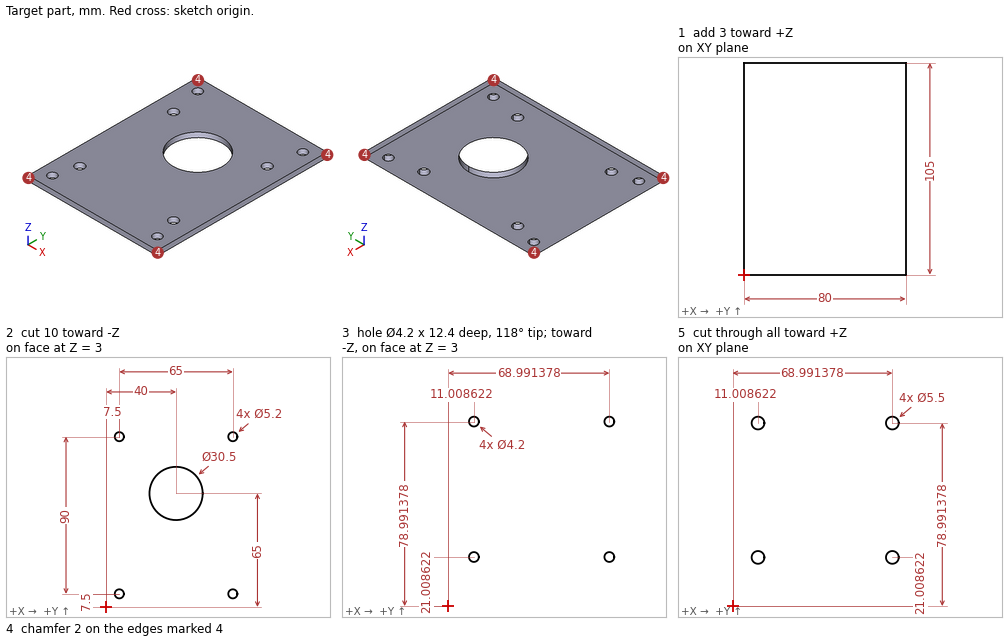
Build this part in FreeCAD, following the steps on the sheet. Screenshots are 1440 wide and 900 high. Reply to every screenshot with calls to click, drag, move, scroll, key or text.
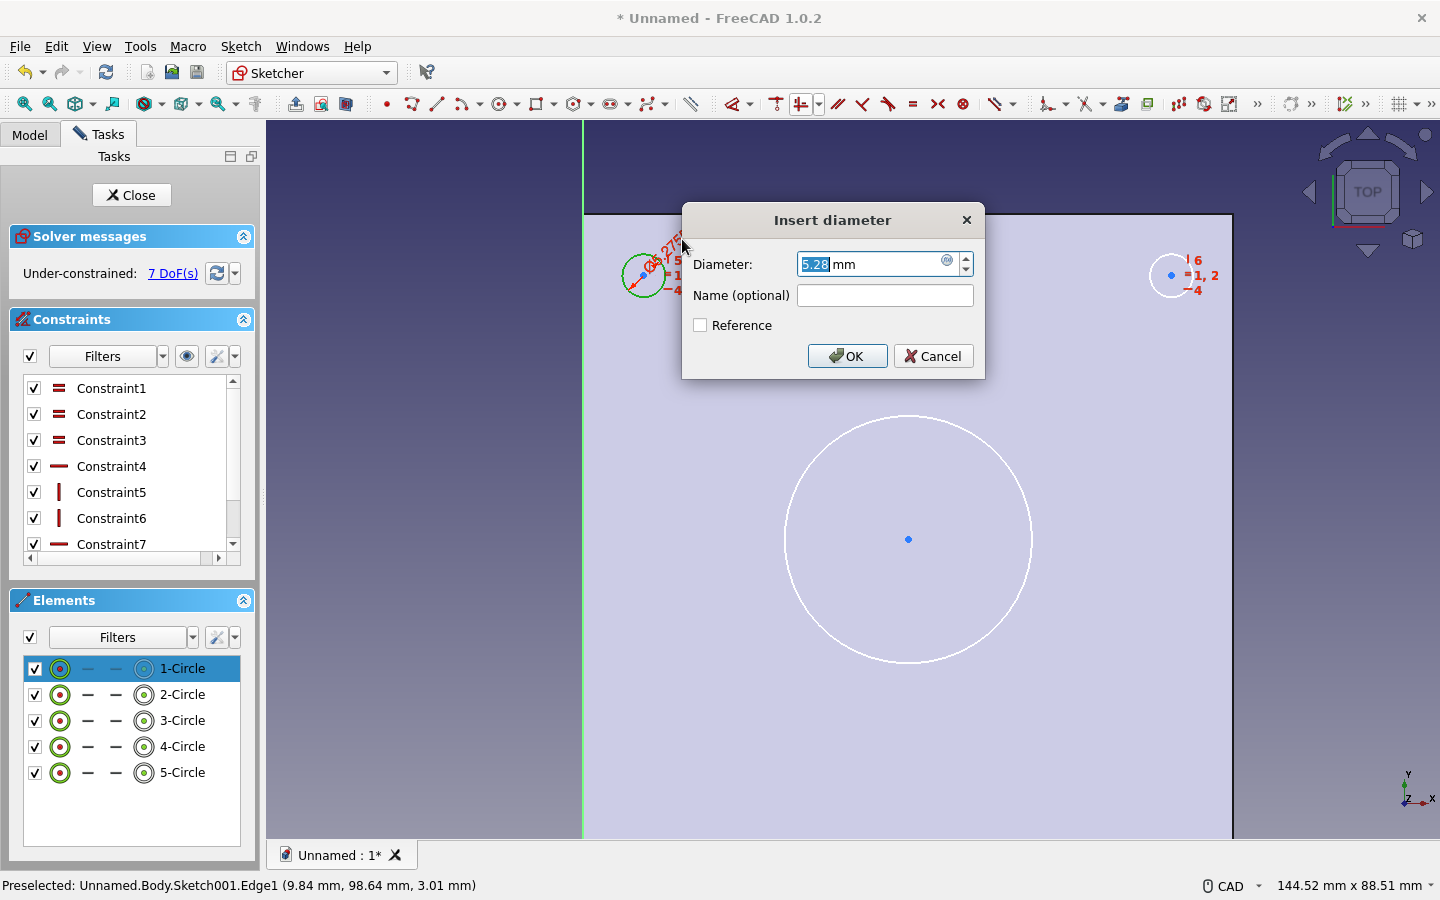
text(5.2)
key(Return)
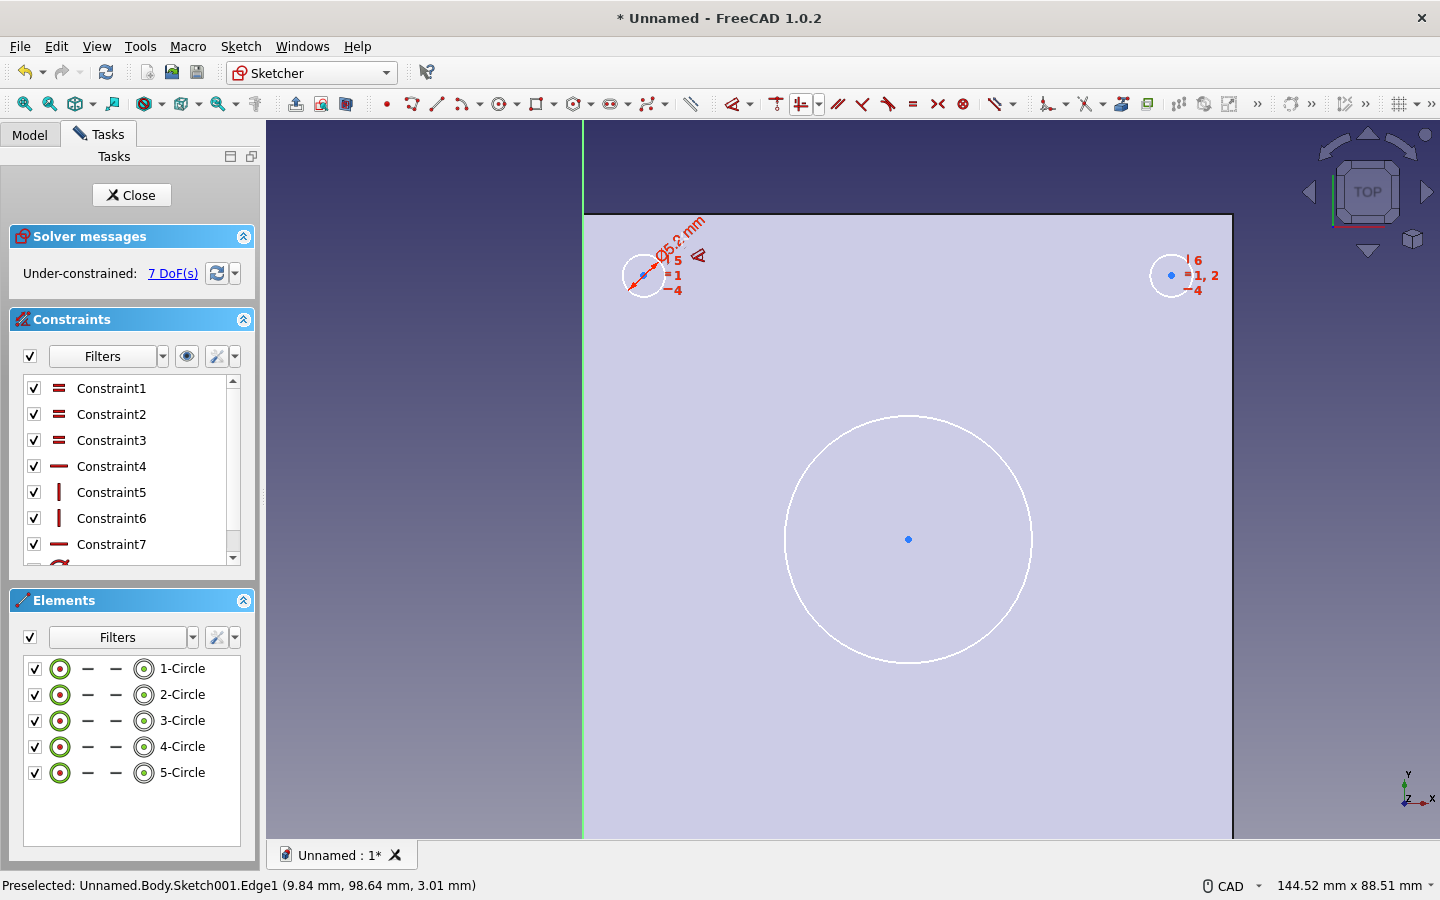
click(996, 452)
click(1019, 429)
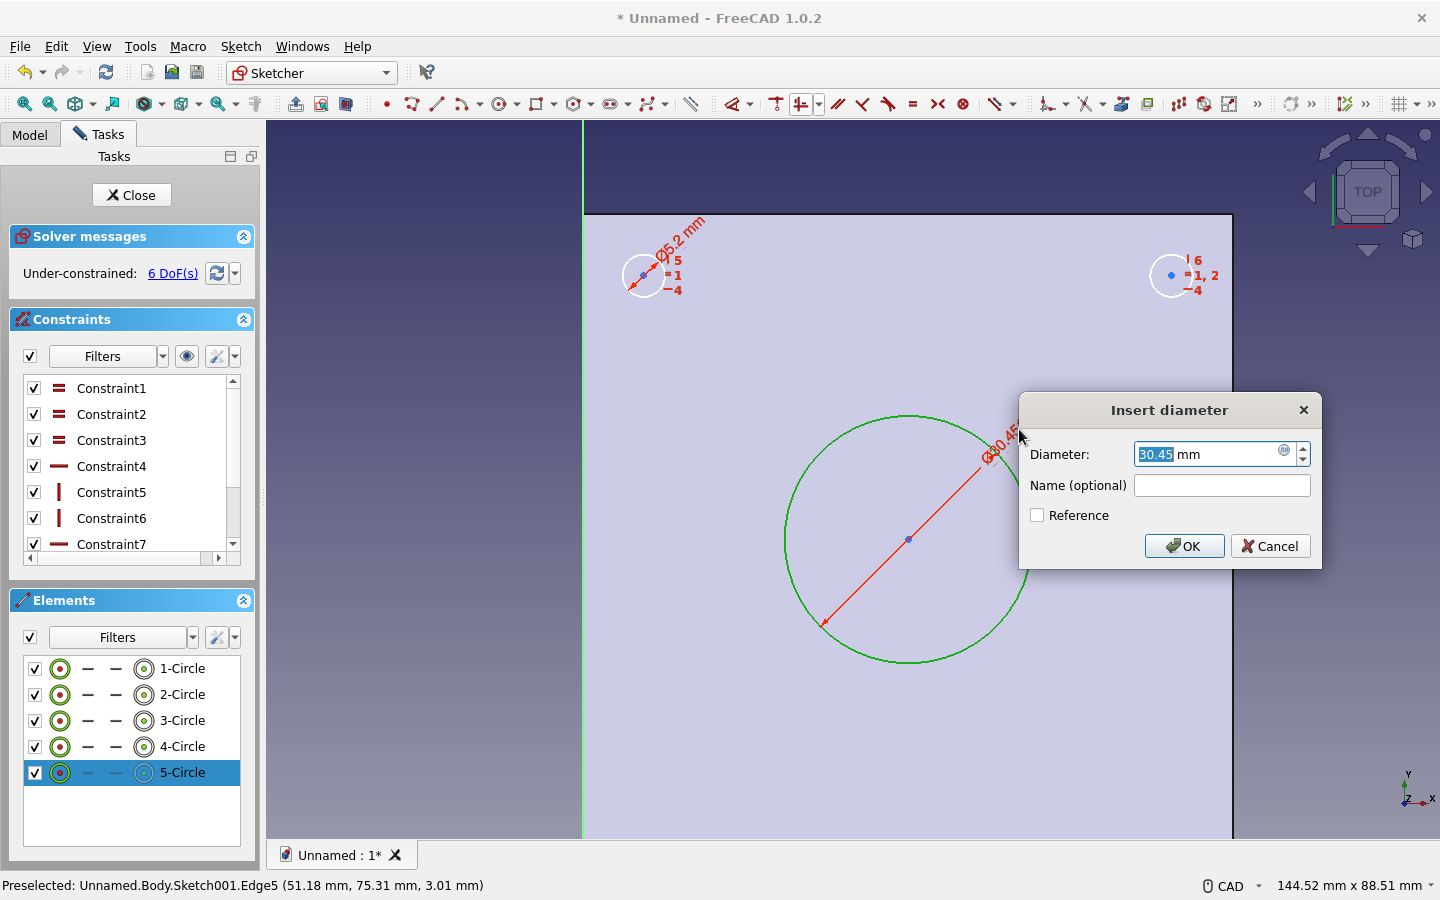
text(30.5)
key(Return)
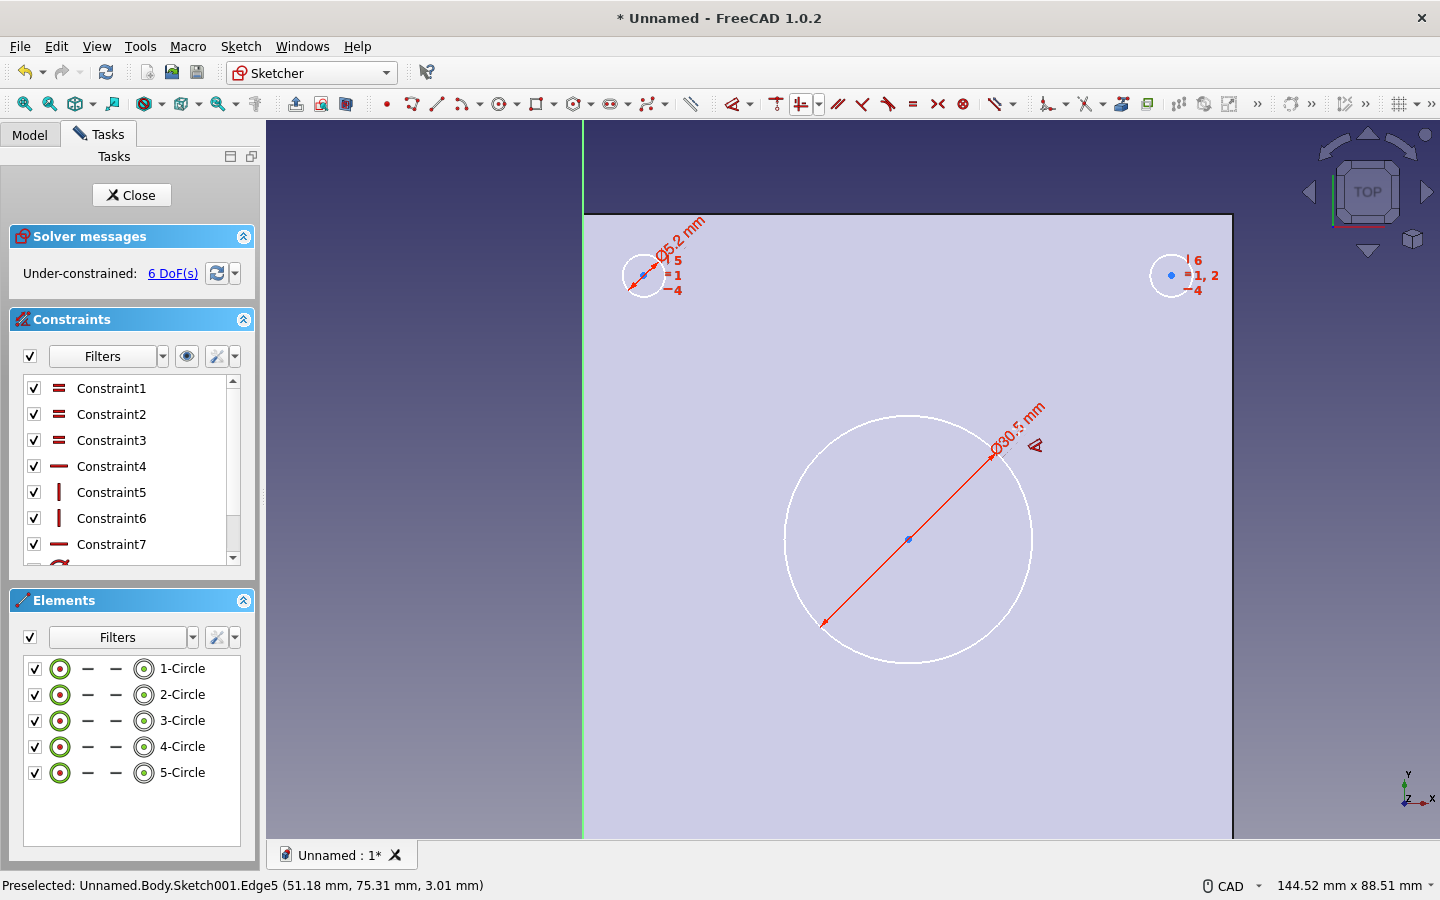
click(908, 540)
click(746, 506)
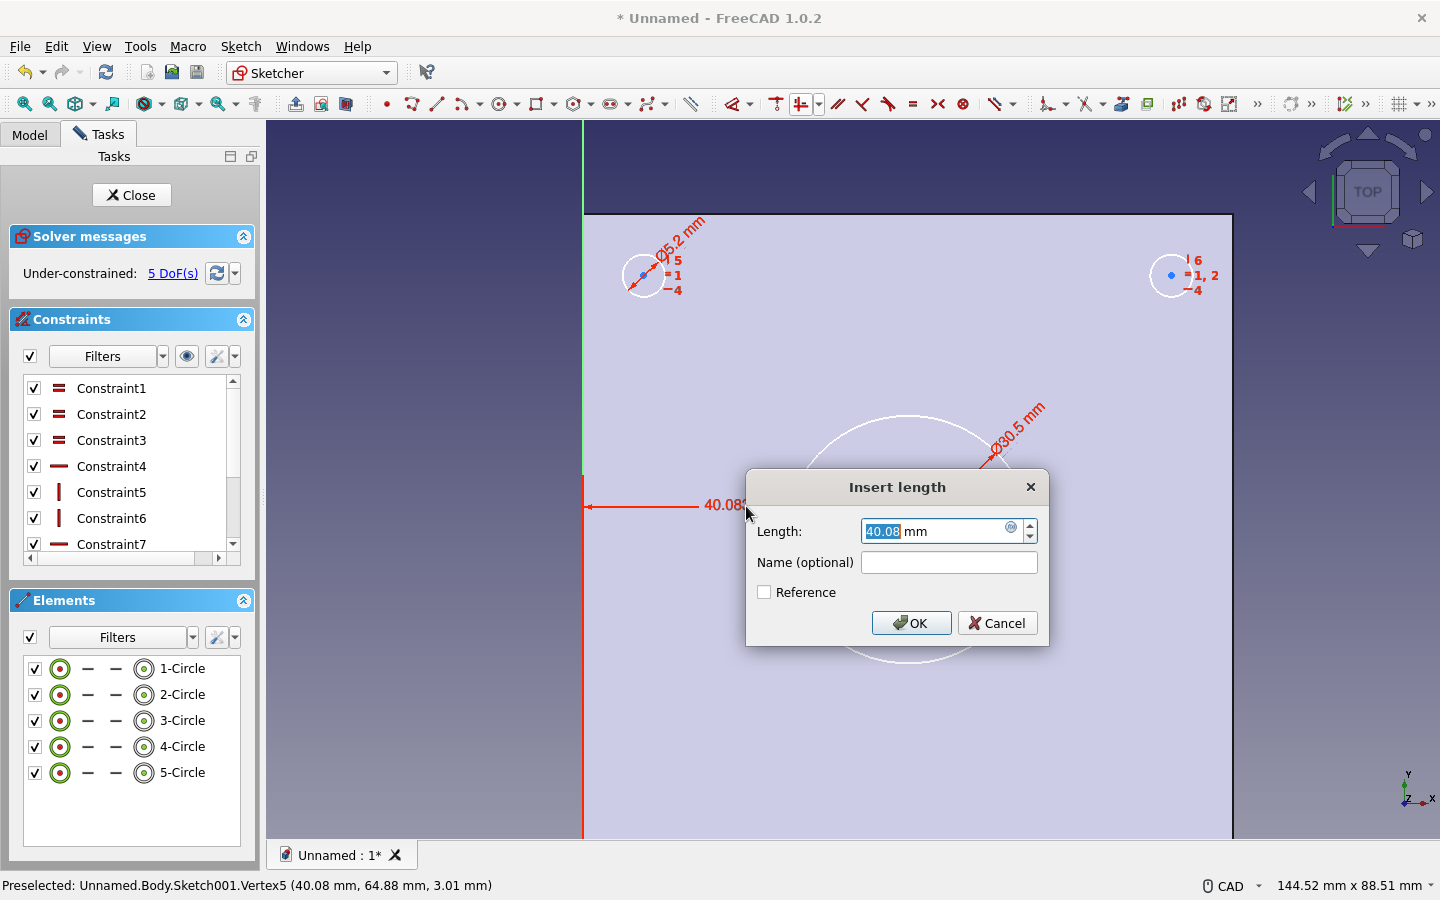
text(40)
key(Return)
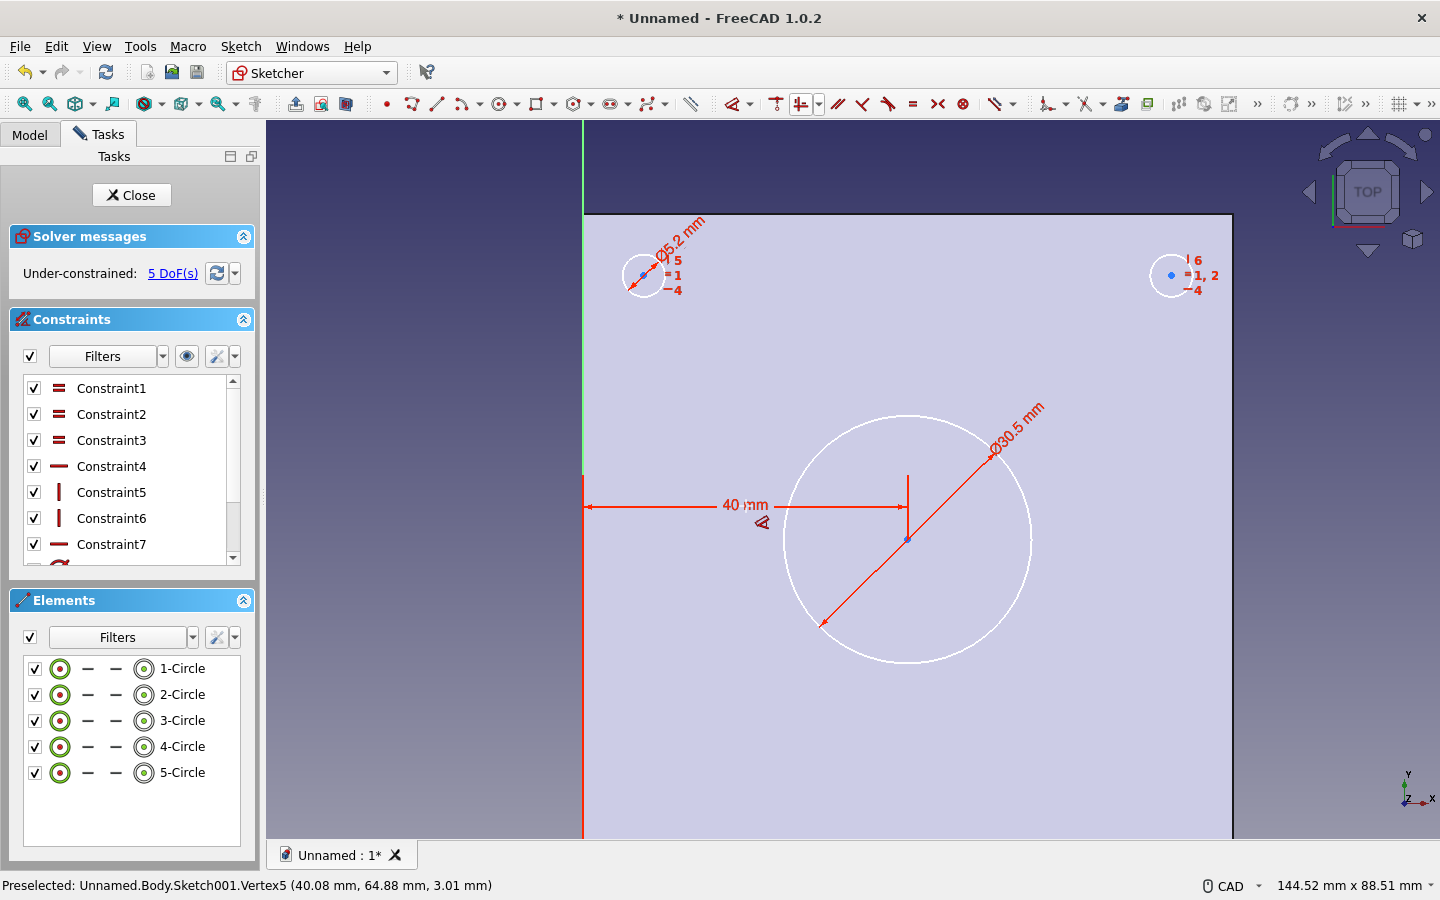
click(908, 540)
click(549, 675)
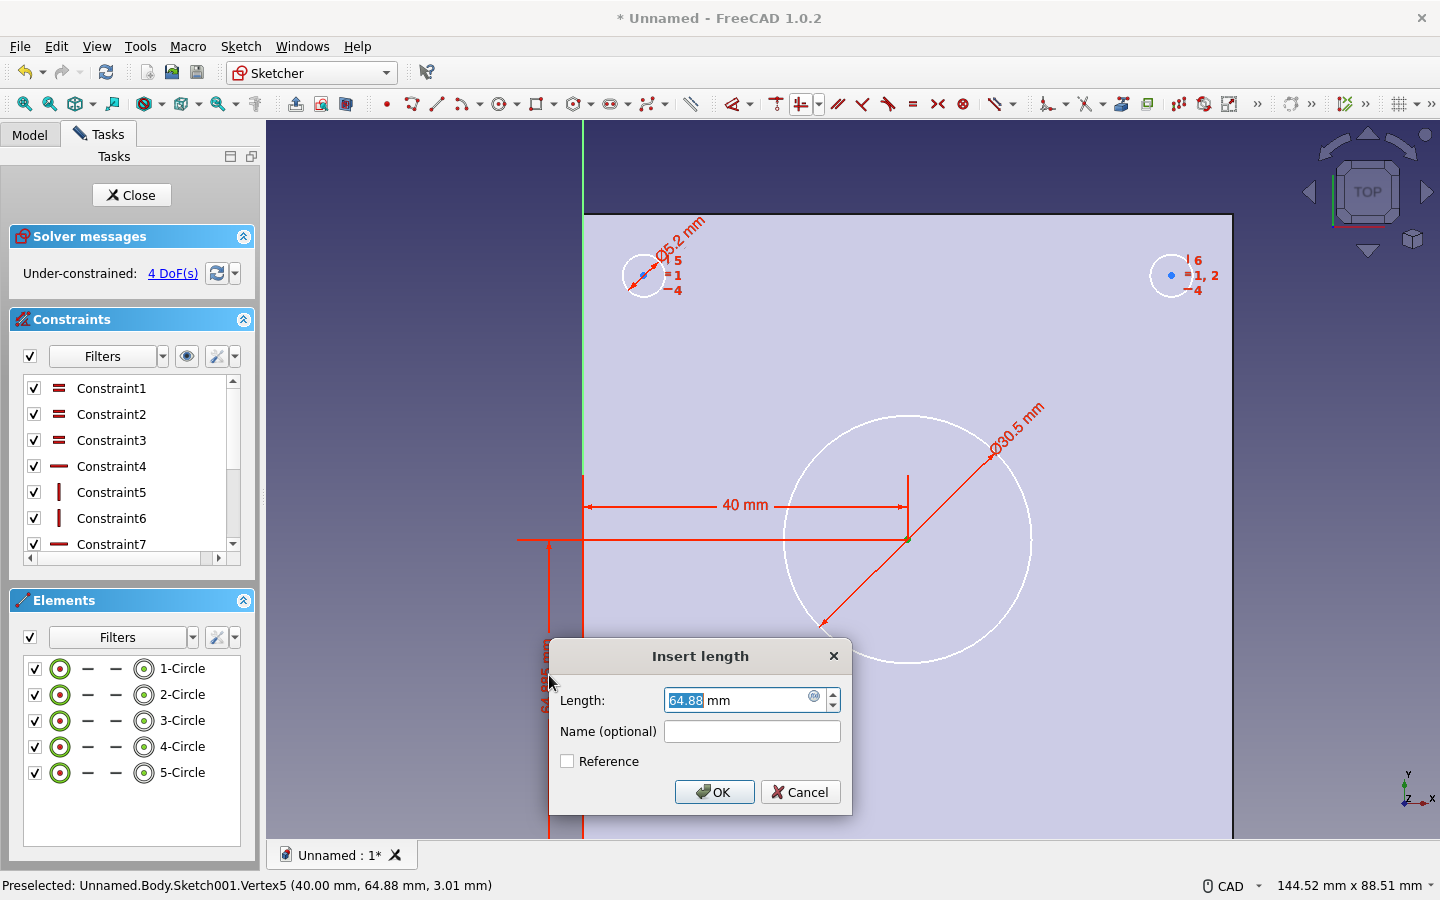
text(65)
key(Return)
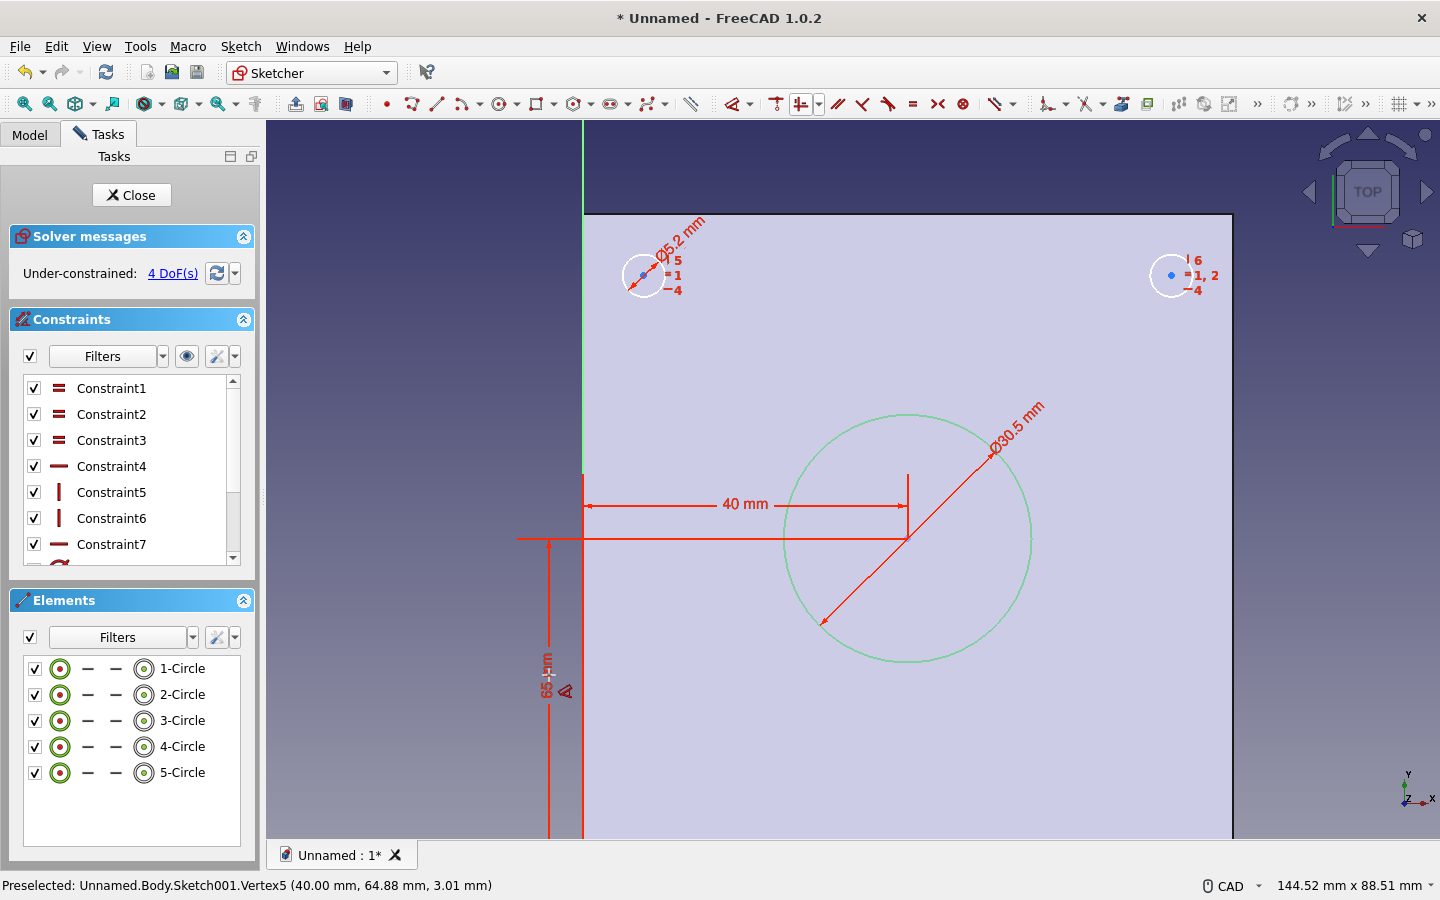
click(644, 276)
click(599, 242)